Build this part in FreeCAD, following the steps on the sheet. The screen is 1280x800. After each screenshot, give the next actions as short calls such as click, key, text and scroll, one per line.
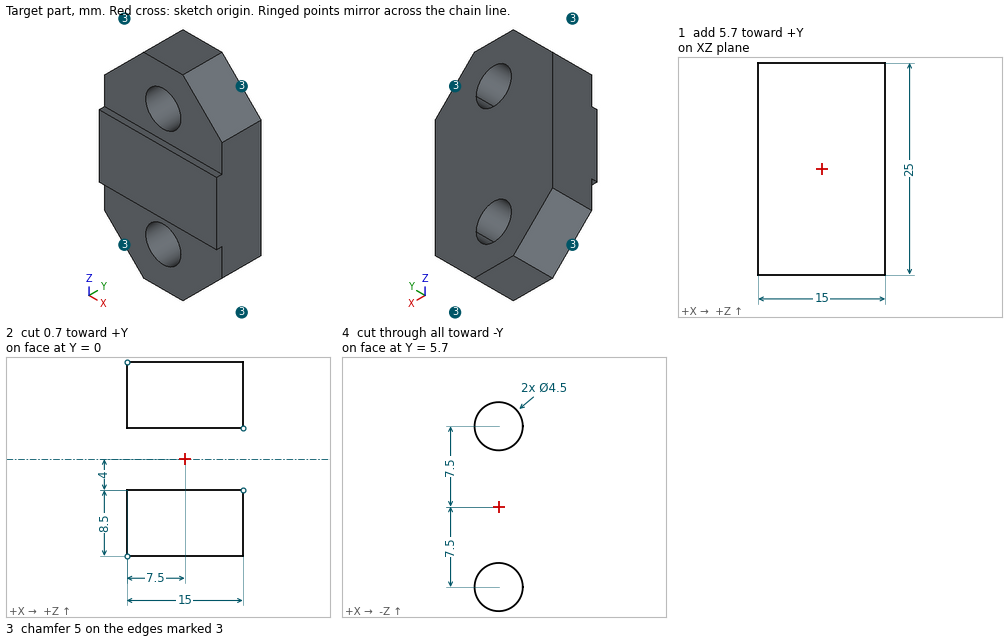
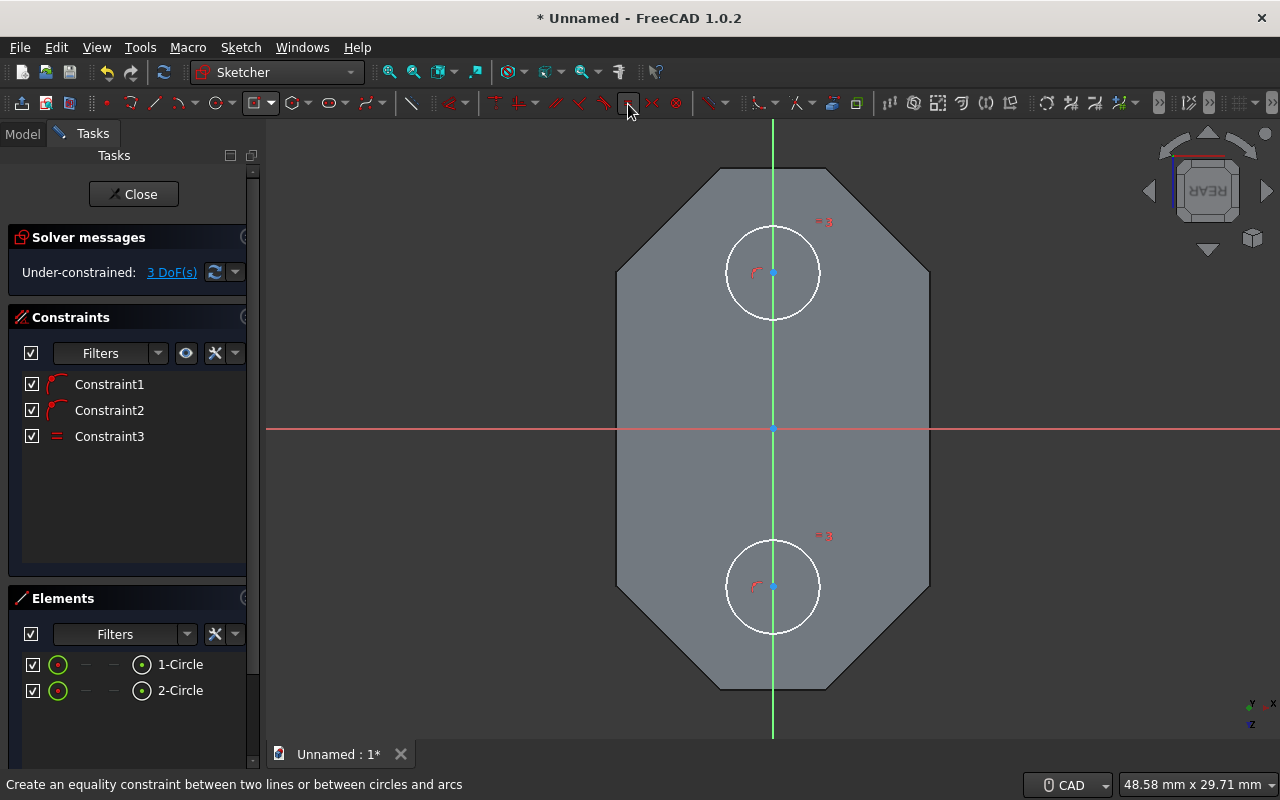
key(d)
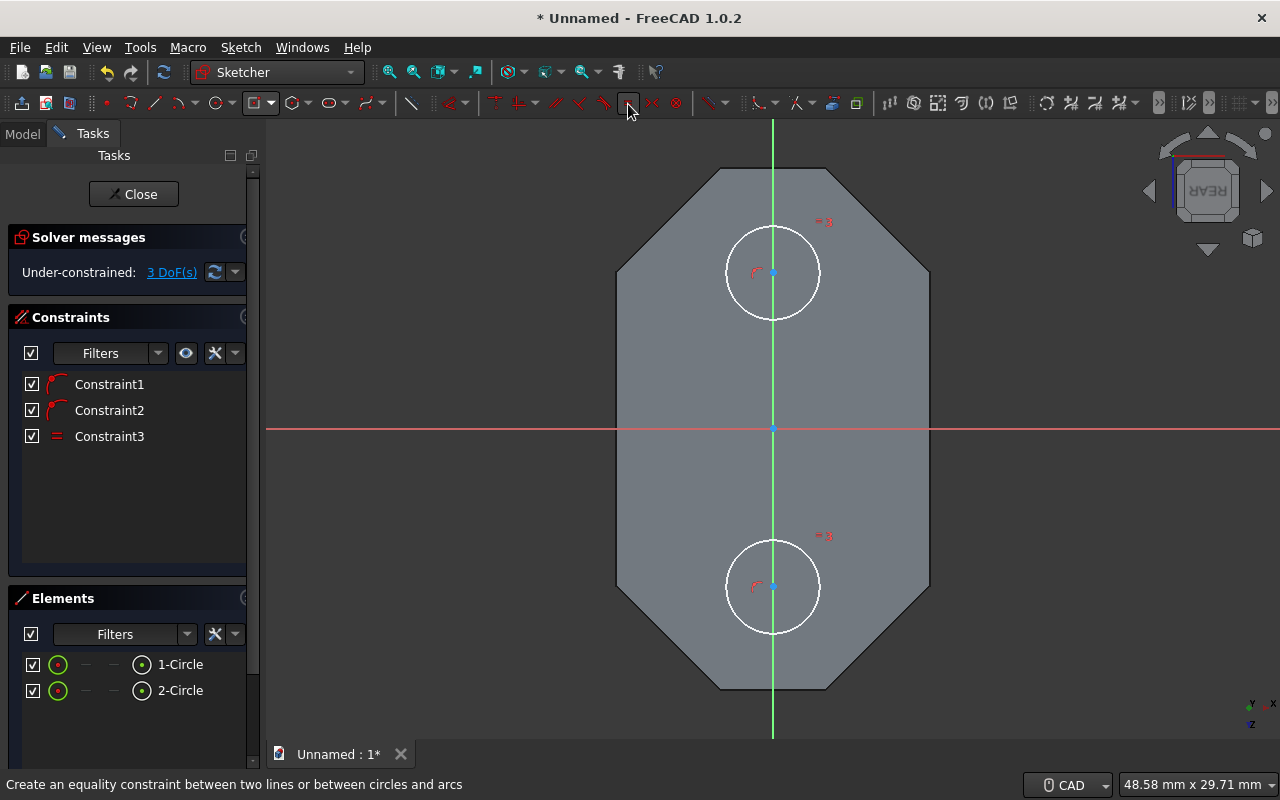
click(806, 240)
click(829, 217)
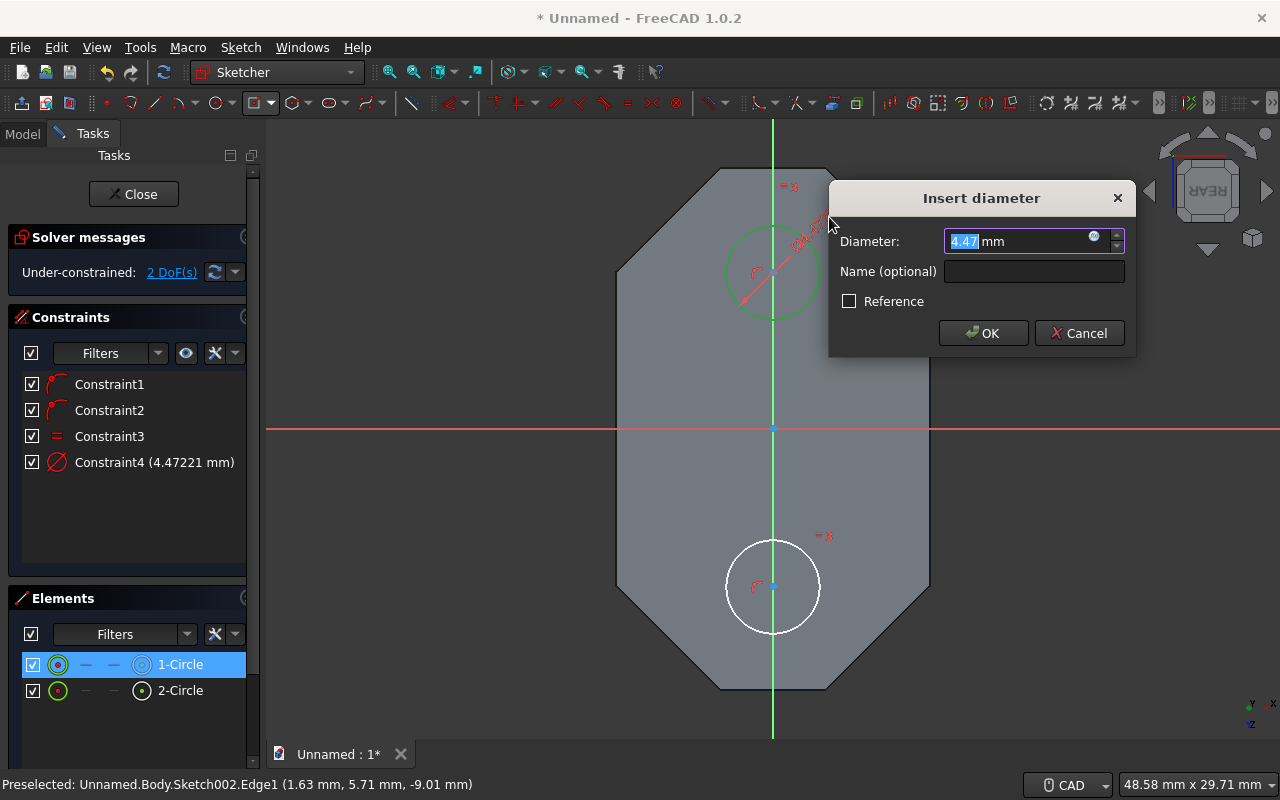
text(4.5)
key(Return)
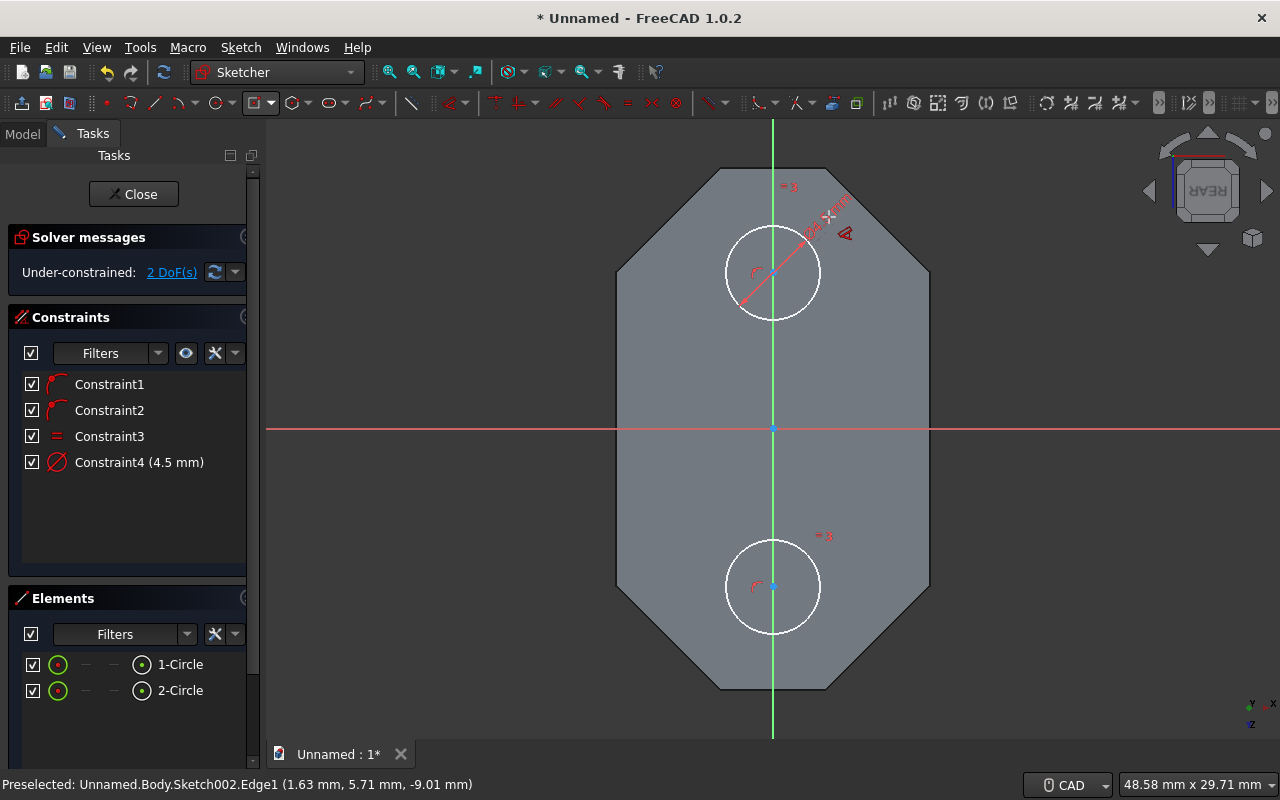
click(773, 273)
click(807, 351)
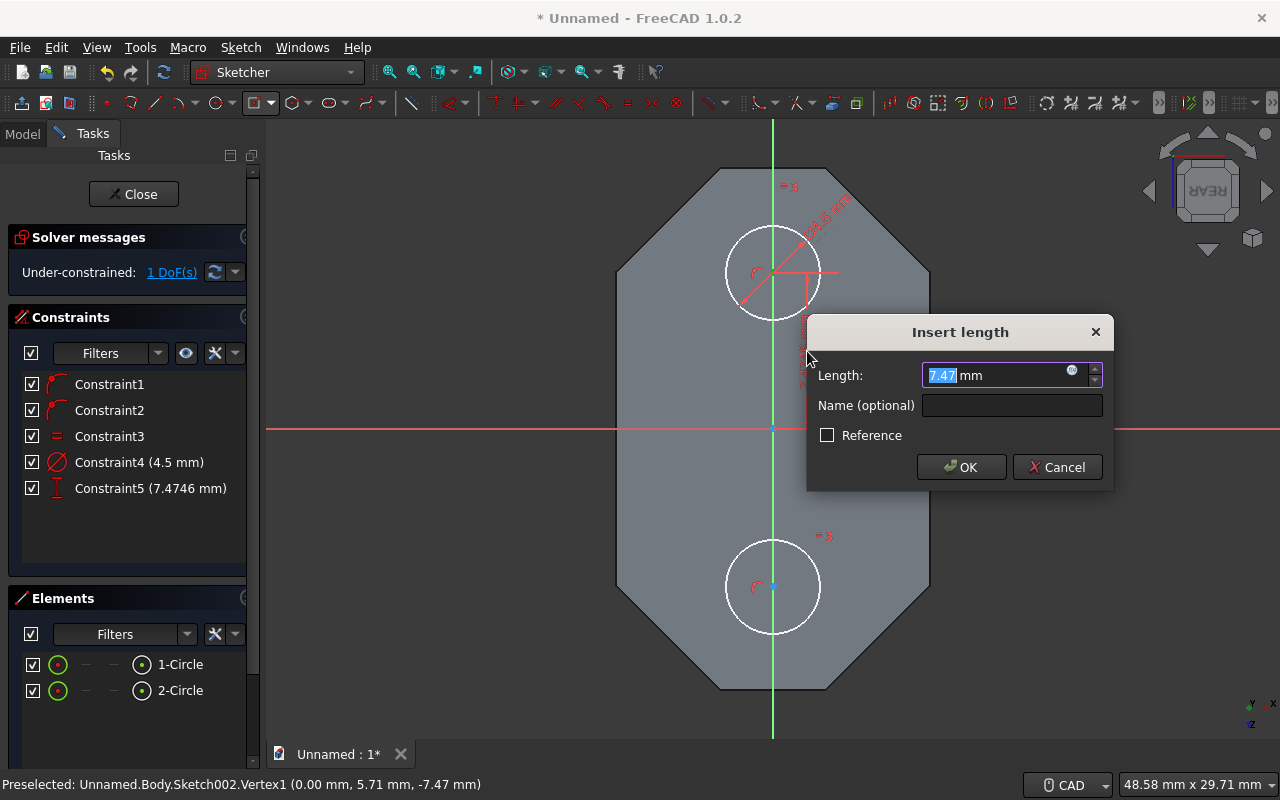
text(7.5)
key(Return)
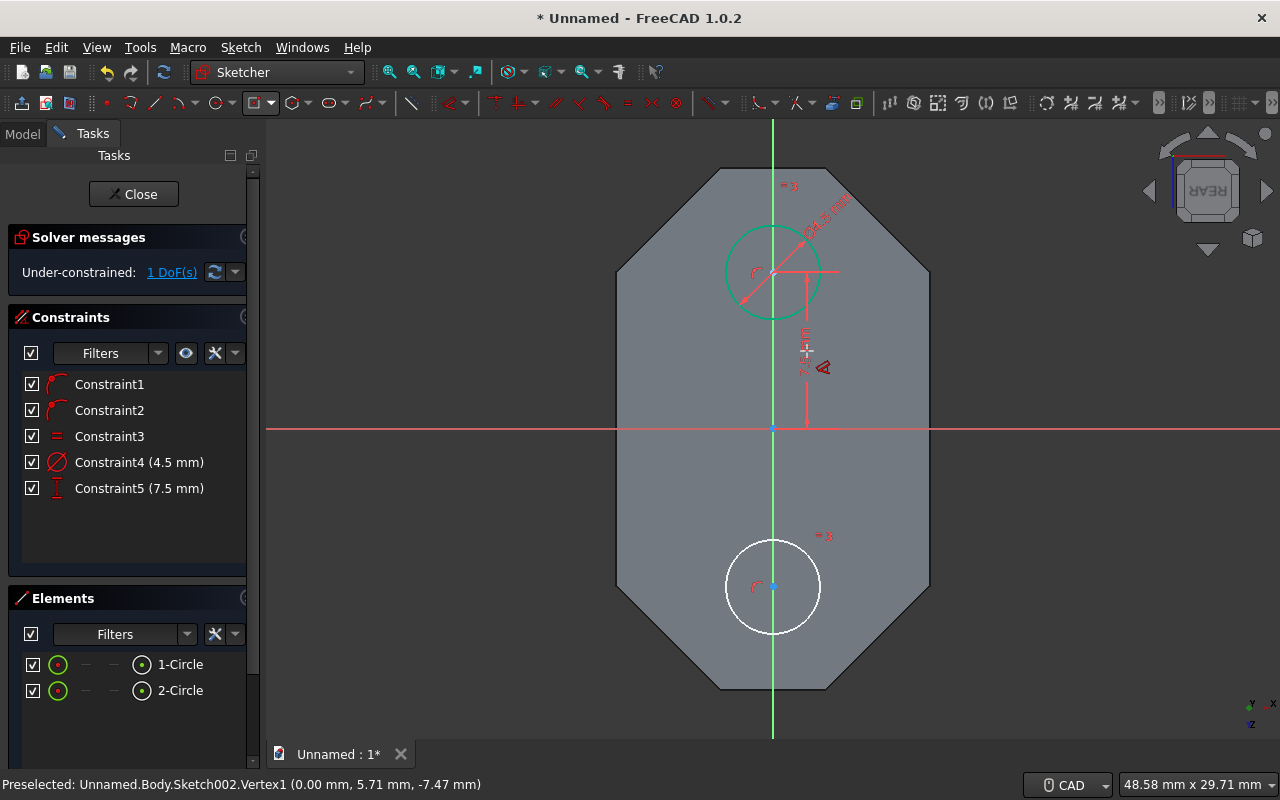
click(773, 587)
click(807, 508)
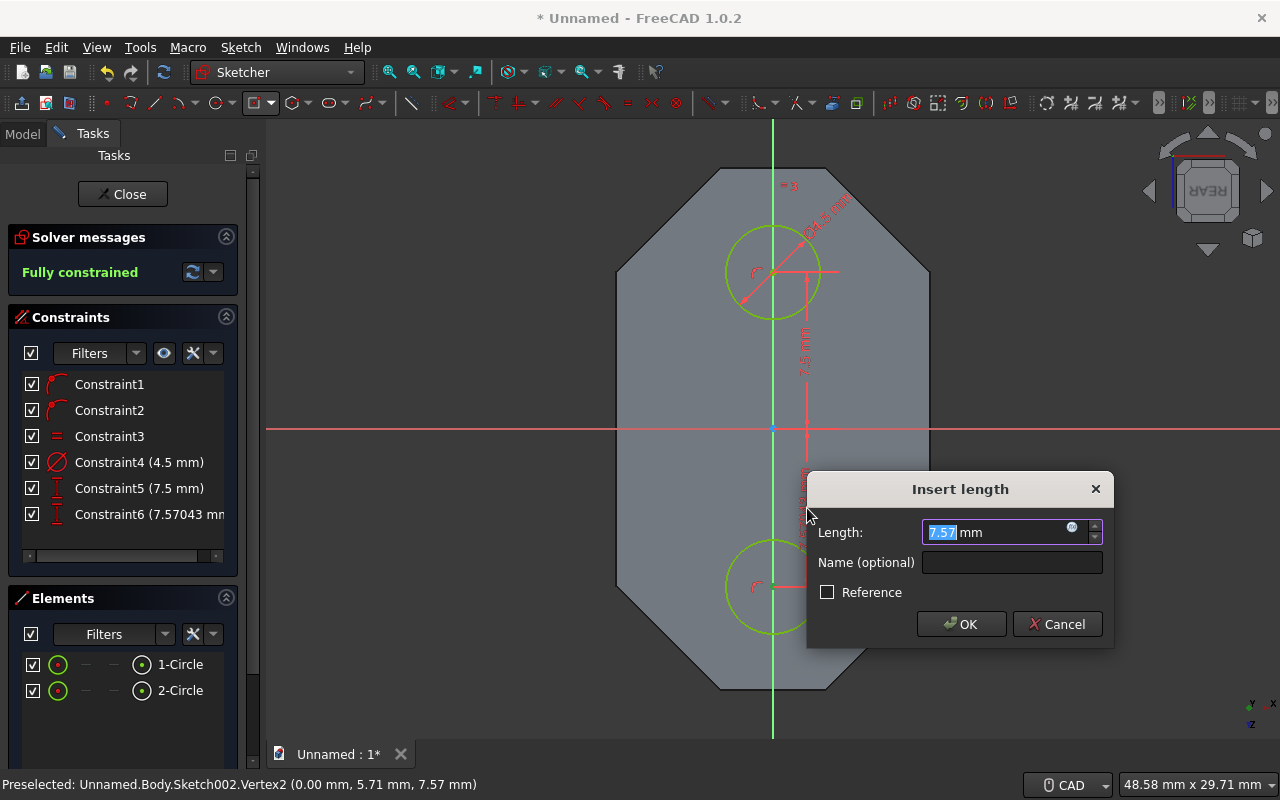
text(7.5)
key(Return)
key(Escape)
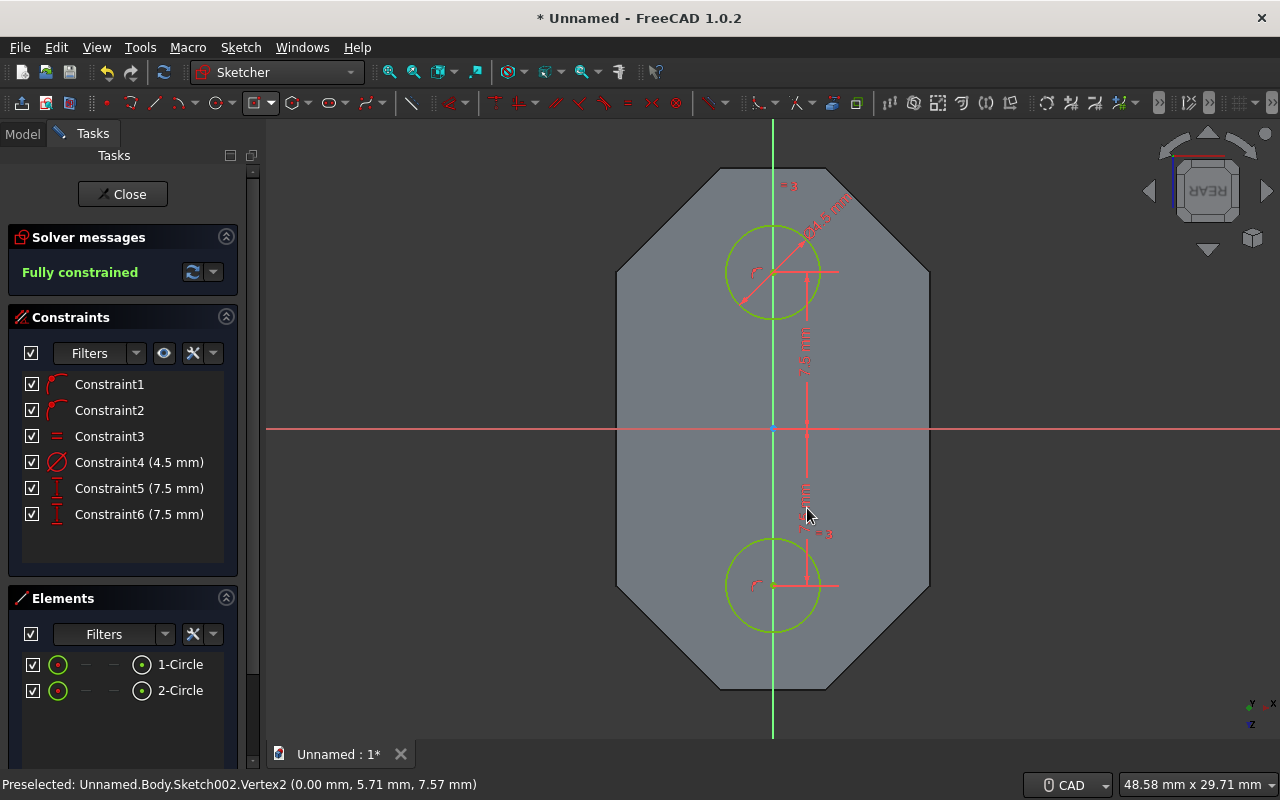
click(123, 194)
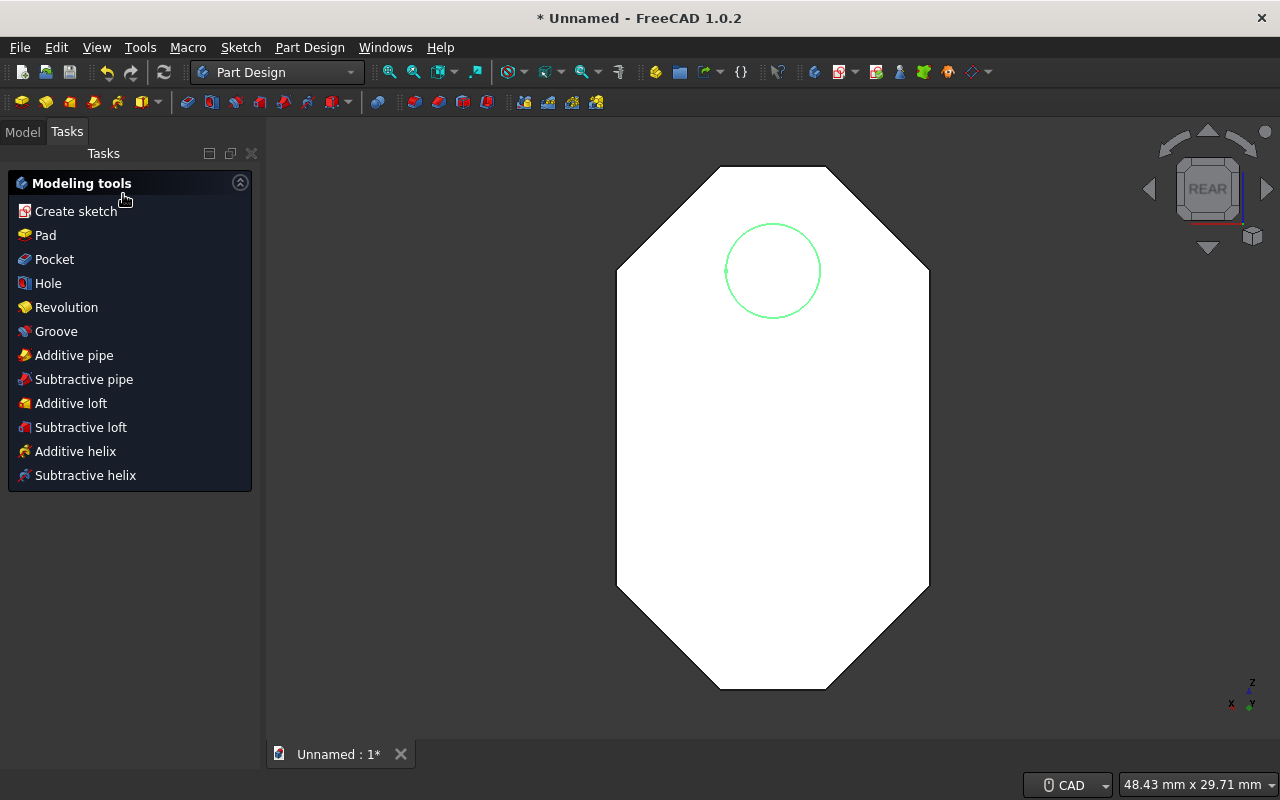
click(188, 102)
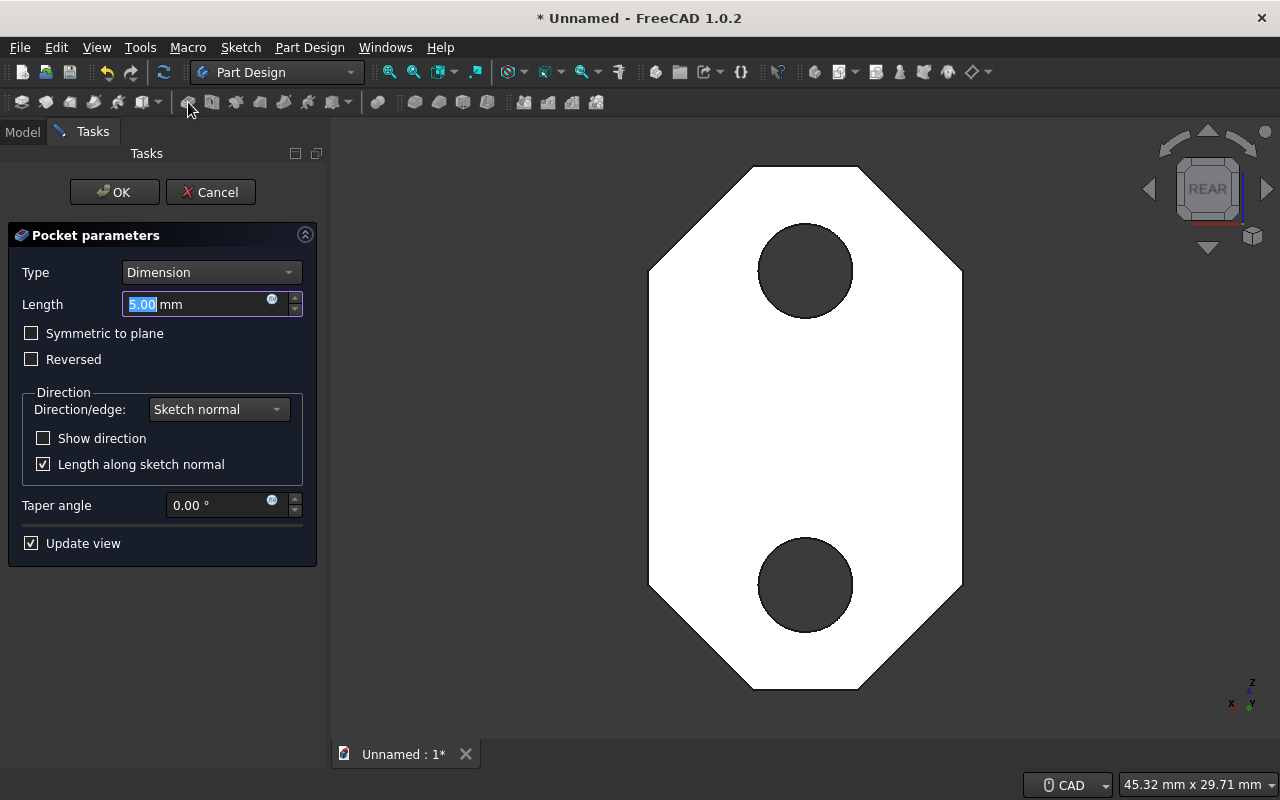
click(212, 272)